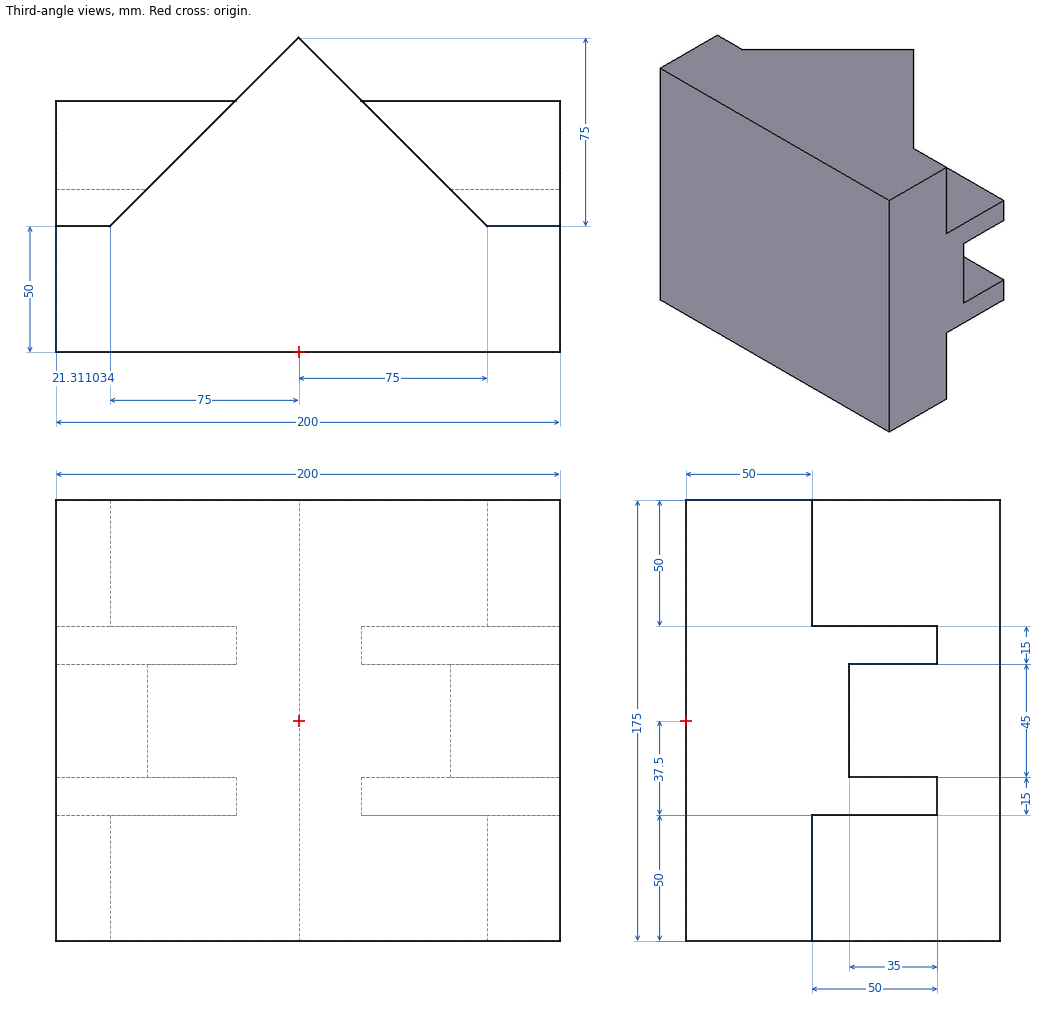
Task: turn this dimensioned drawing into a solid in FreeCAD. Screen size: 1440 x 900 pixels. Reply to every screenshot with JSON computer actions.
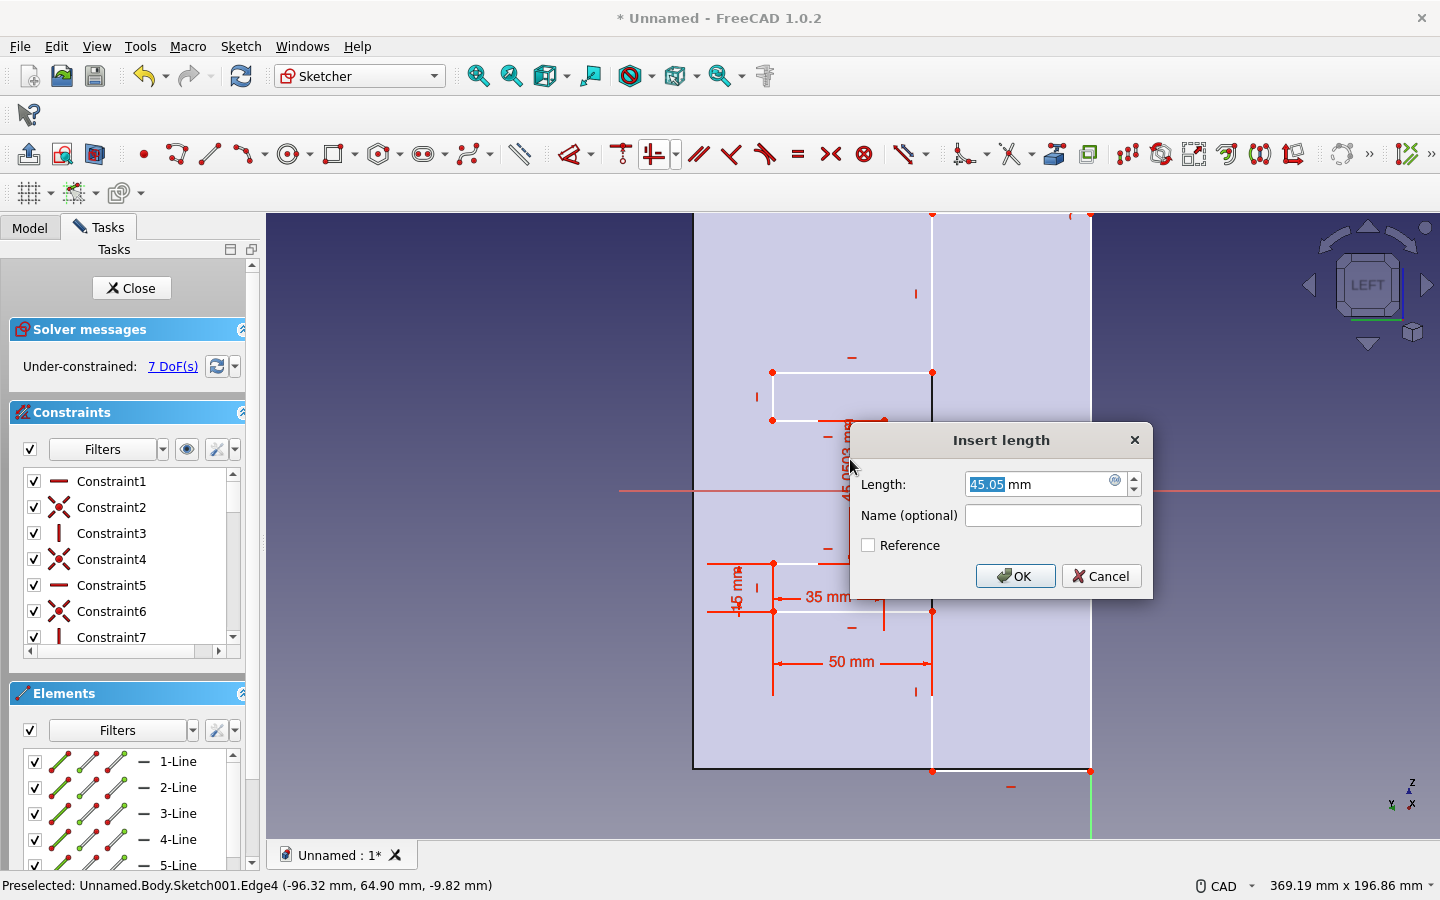
{"action": "type", "text": "45"}
{"action": "key", "text": "Return"}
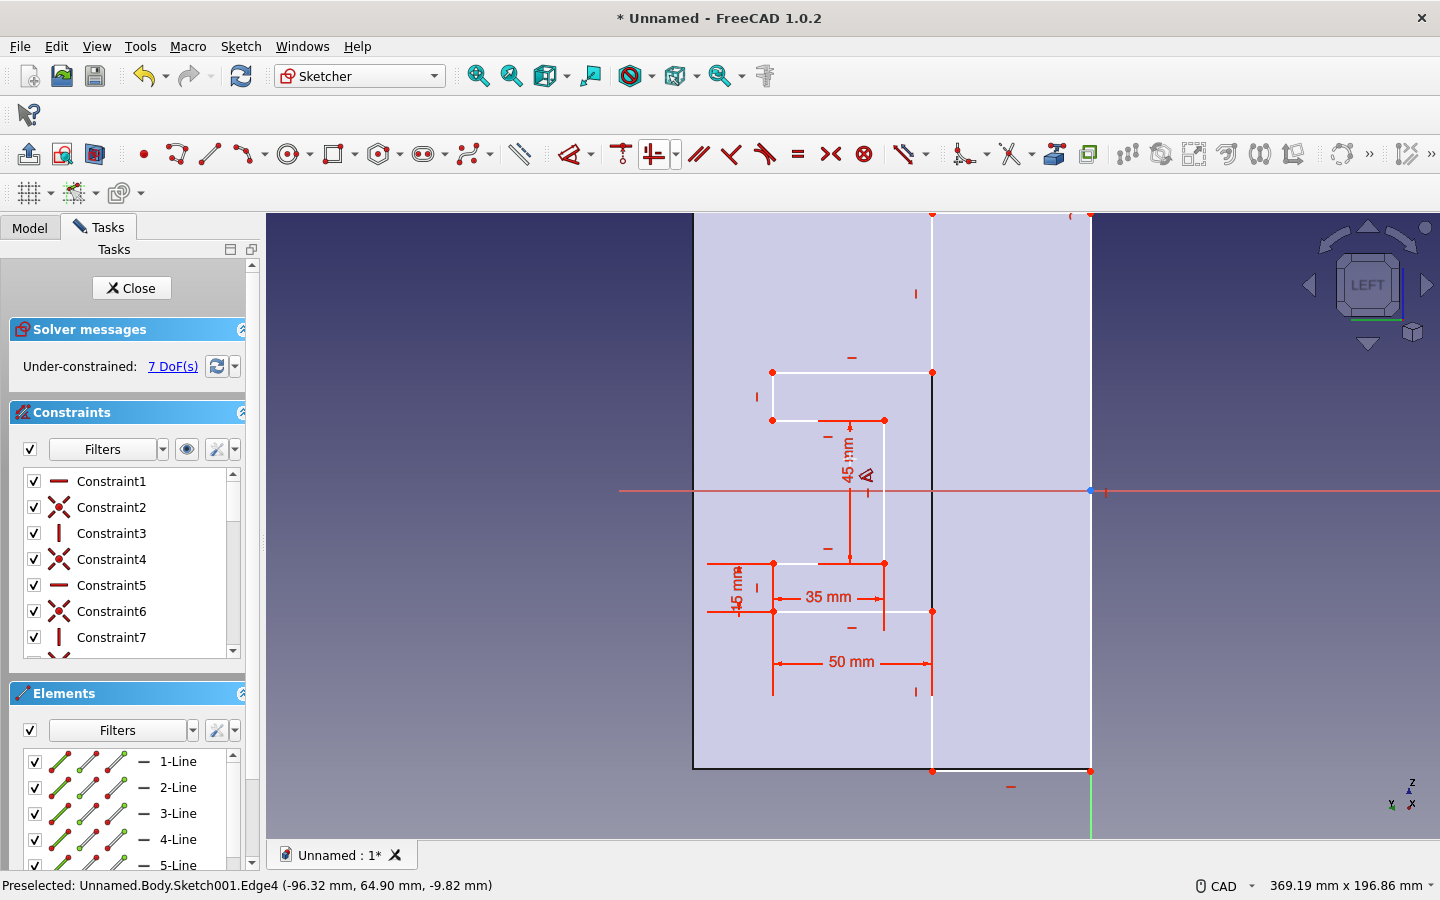
{"action": "left_click", "coordinate": [851, 421]}
{"action": "left_click", "coordinate": [829, 387]}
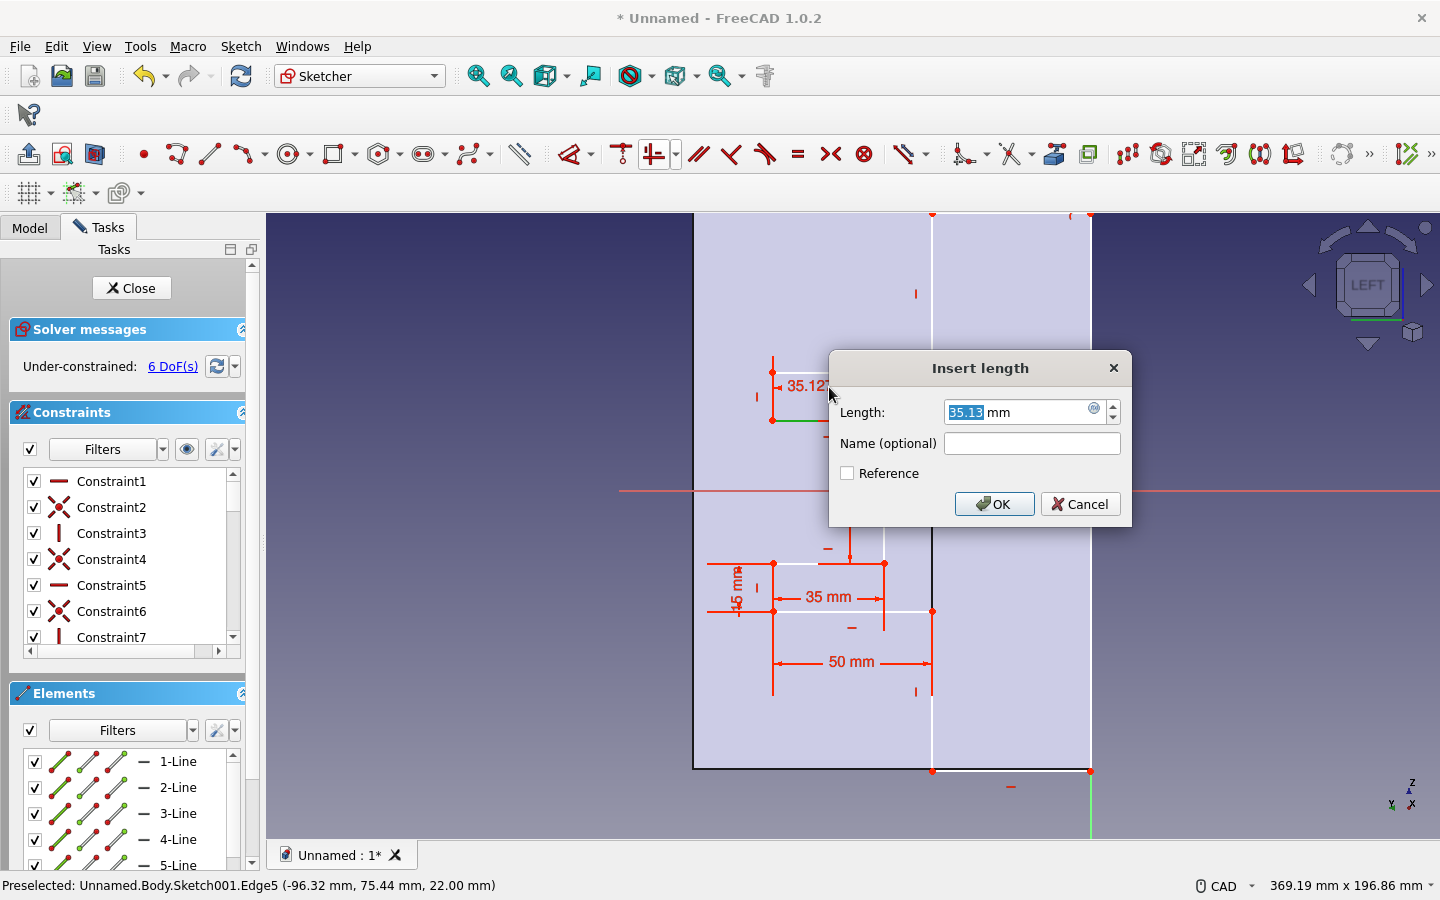
{"action": "type", "text": "35"}
{"action": "key", "text": "Return"}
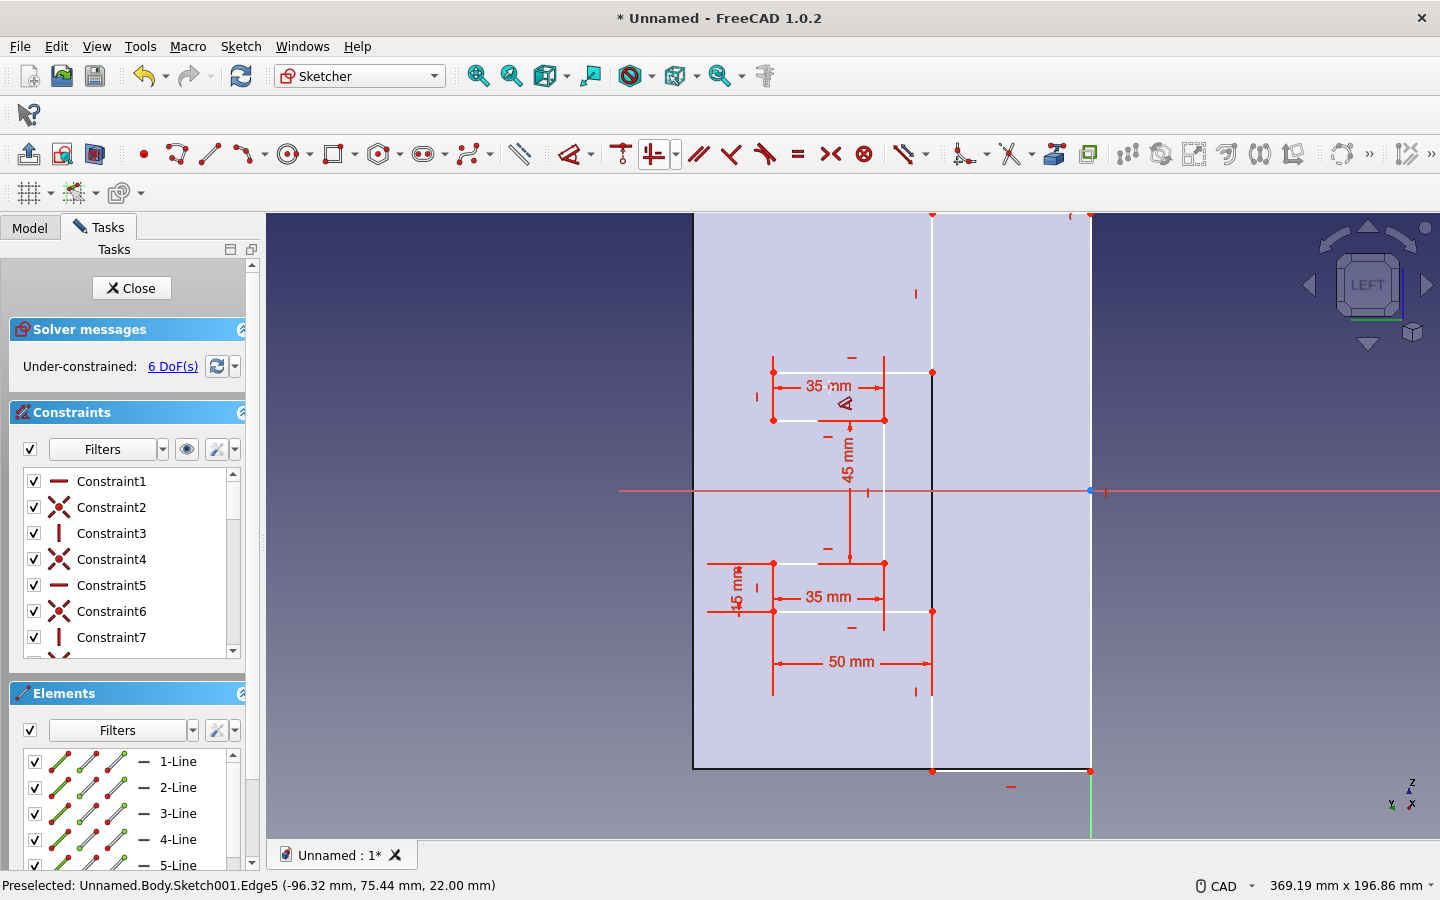
{"action": "left_click", "coordinate": [773, 406]}
{"action": "left_click", "coordinate": [739, 397]}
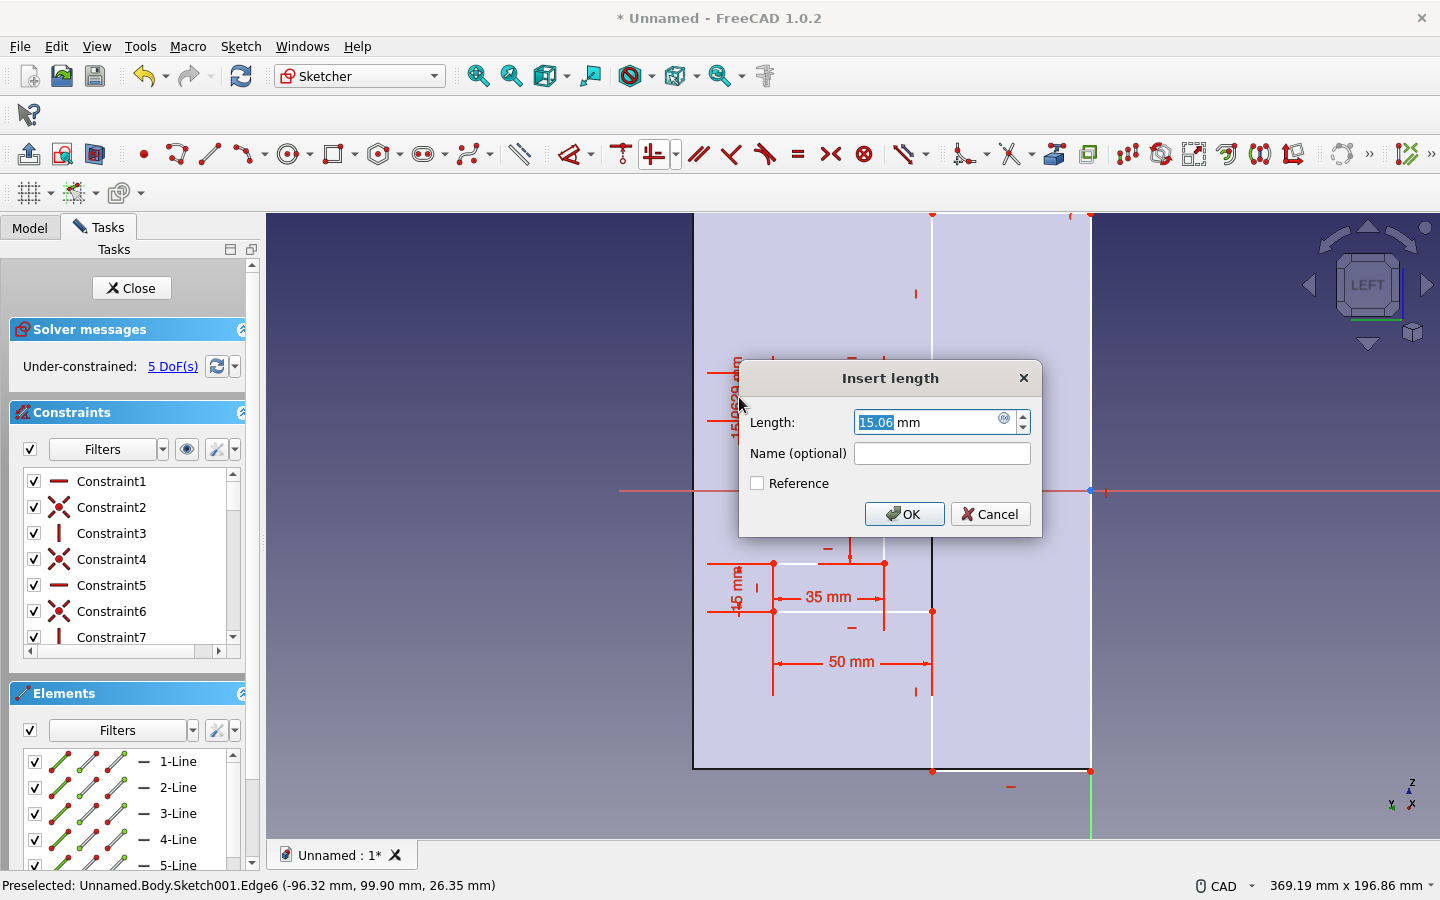
{"action": "type", "text": "15"}
{"action": "key", "text": "Return"}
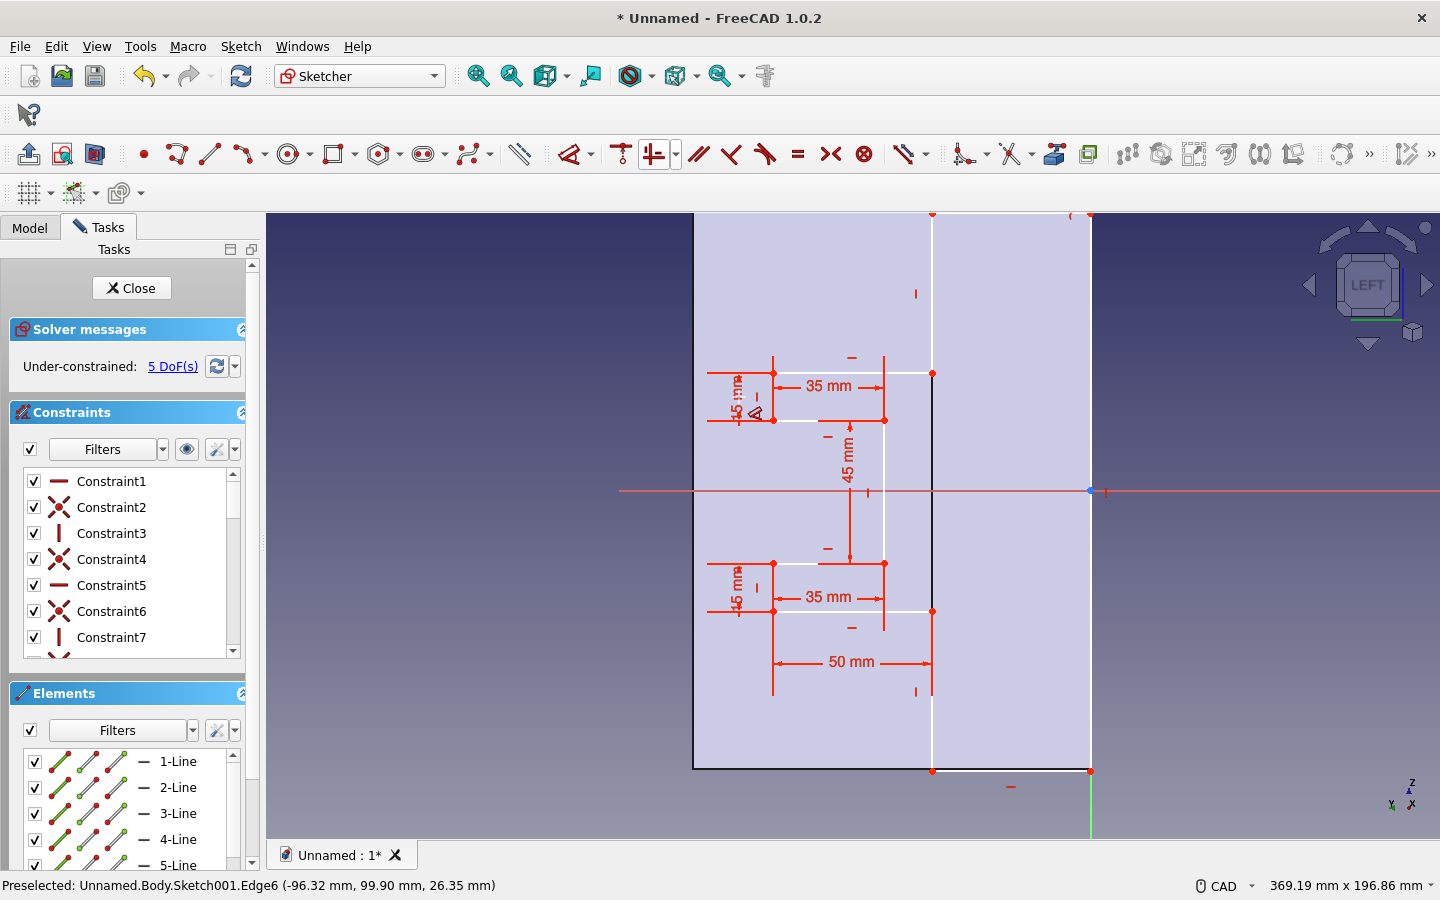
{"action": "left_click", "coordinate": [821, 373]}
{"action": "left_click", "coordinate": [853, 339]}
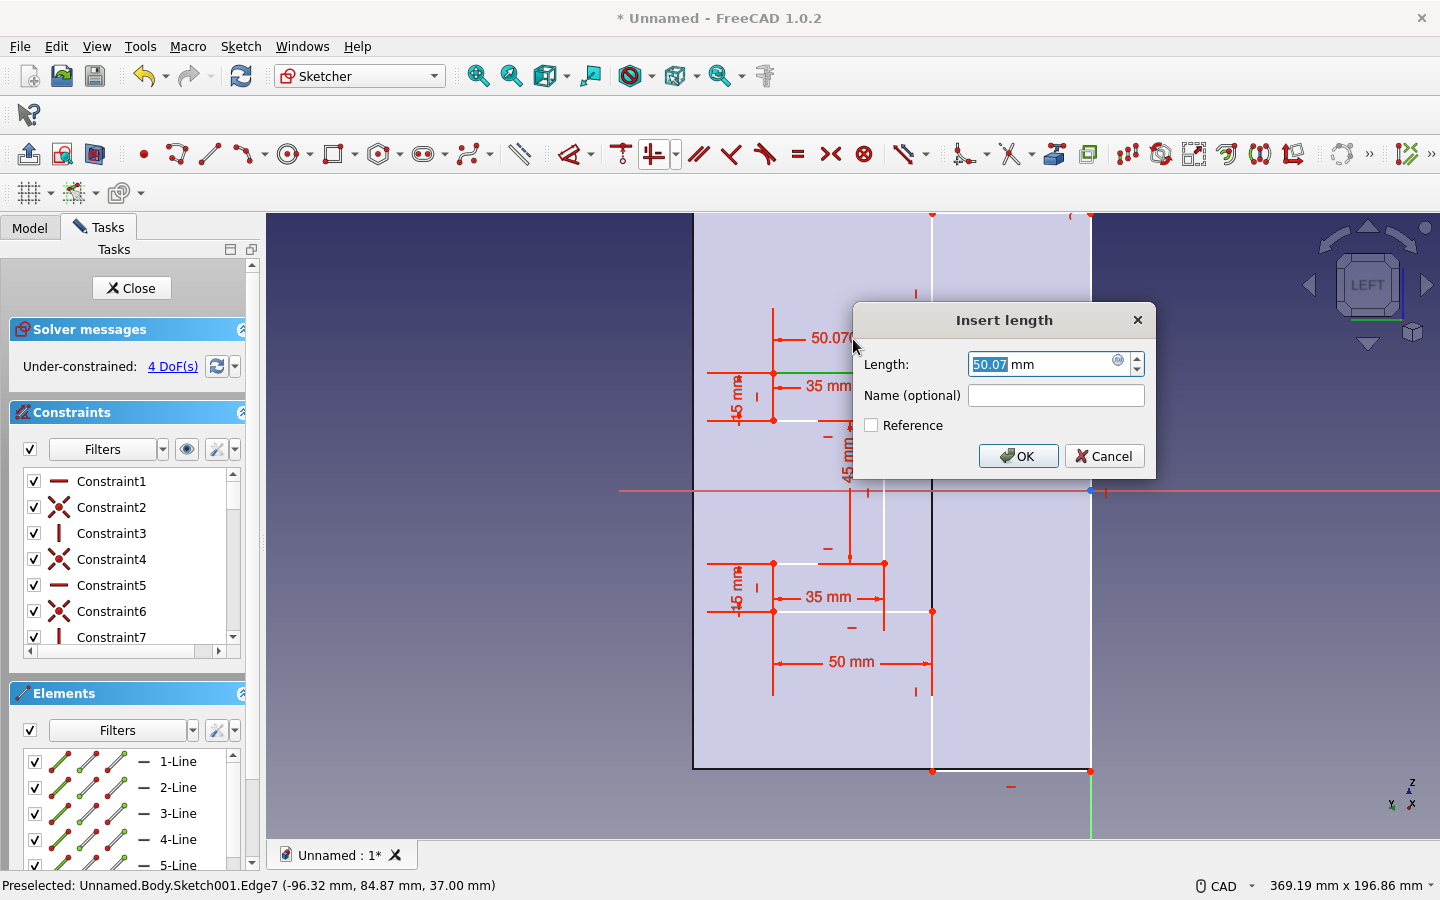
{"action": "type", "text": "50"}
{"action": "key", "text": "Return"}